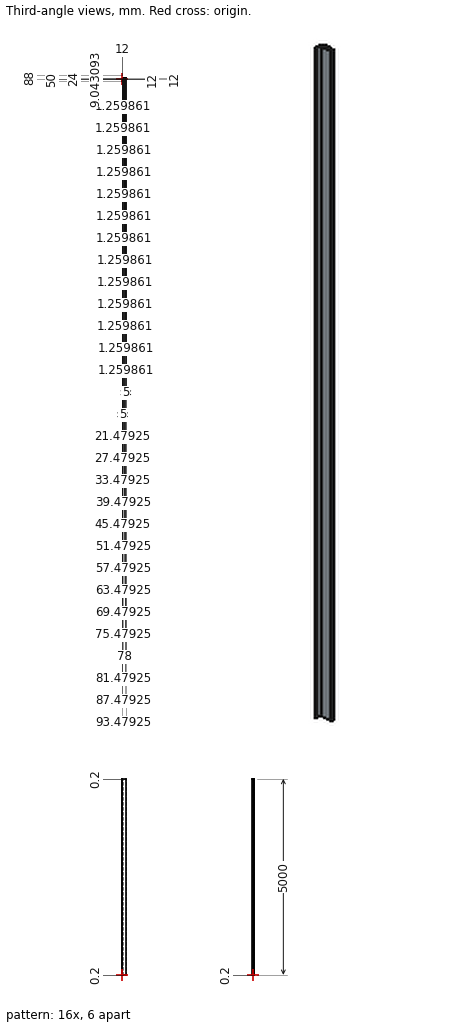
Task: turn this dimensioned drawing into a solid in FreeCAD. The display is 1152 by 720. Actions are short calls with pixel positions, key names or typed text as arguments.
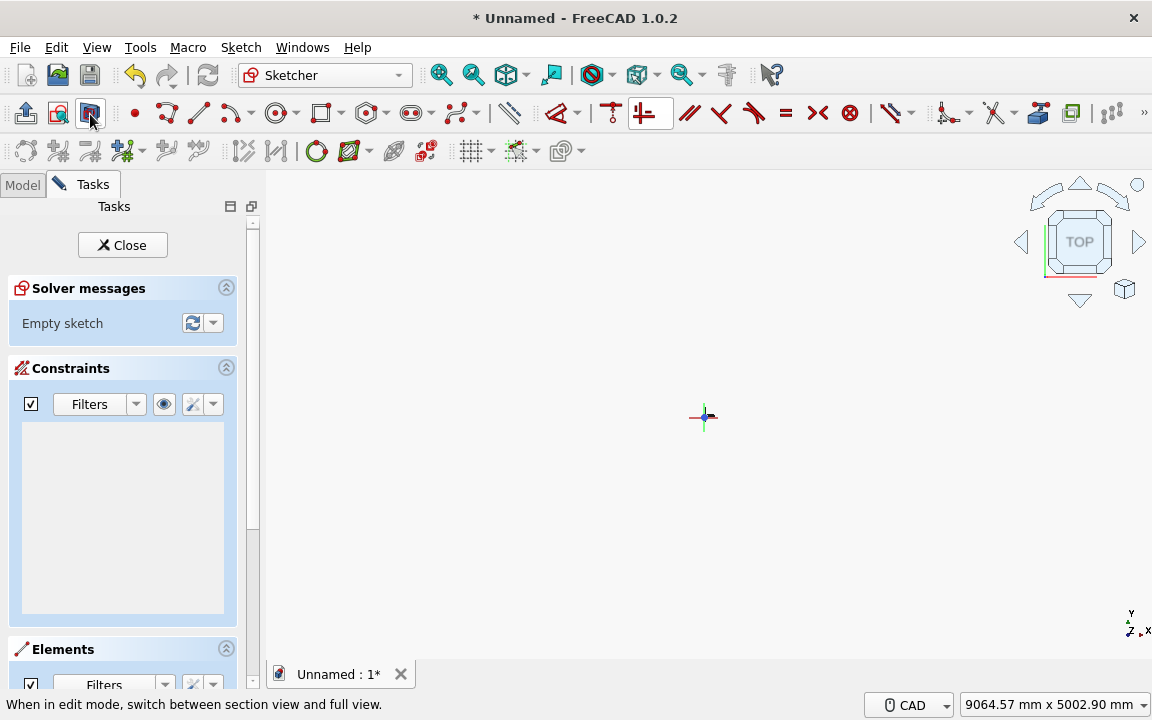
scroll(708, 413, up, 15)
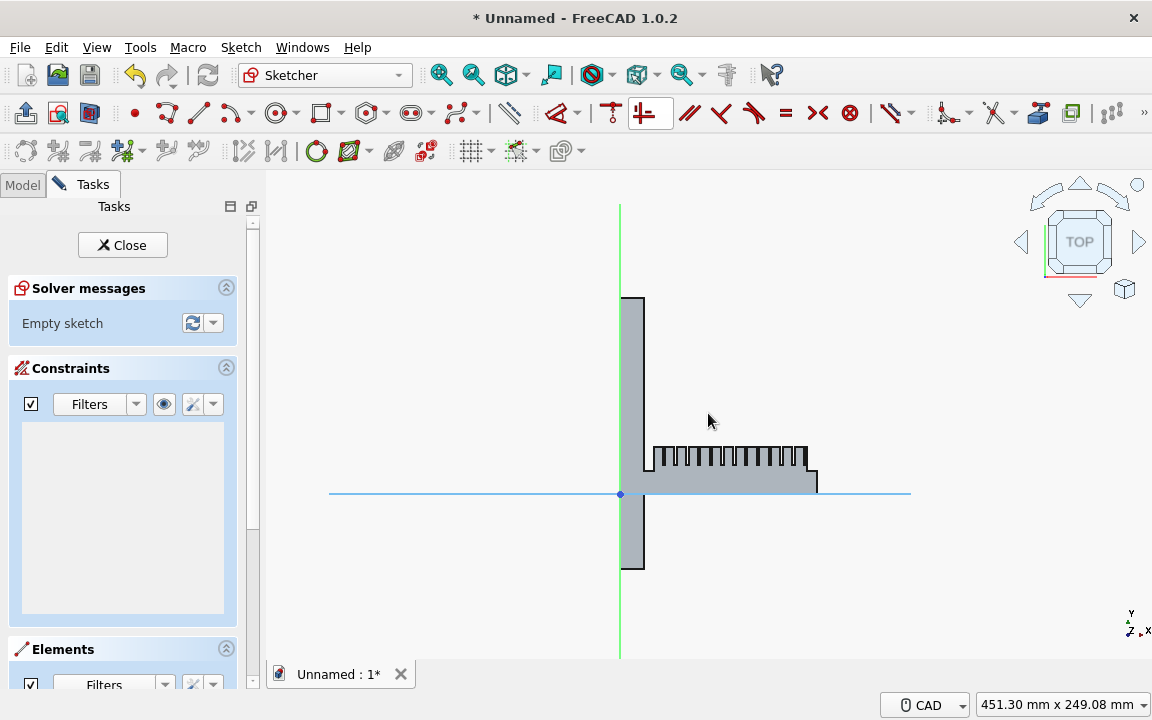
scroll(615, 359, up, 2)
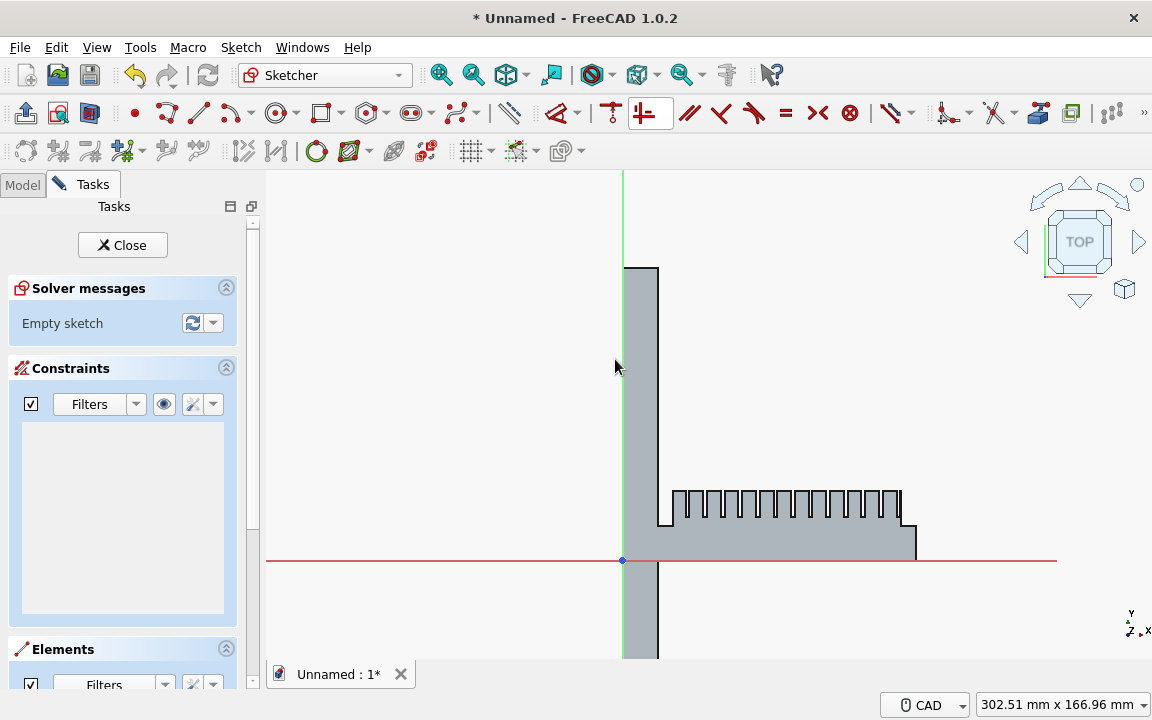
click(322, 114)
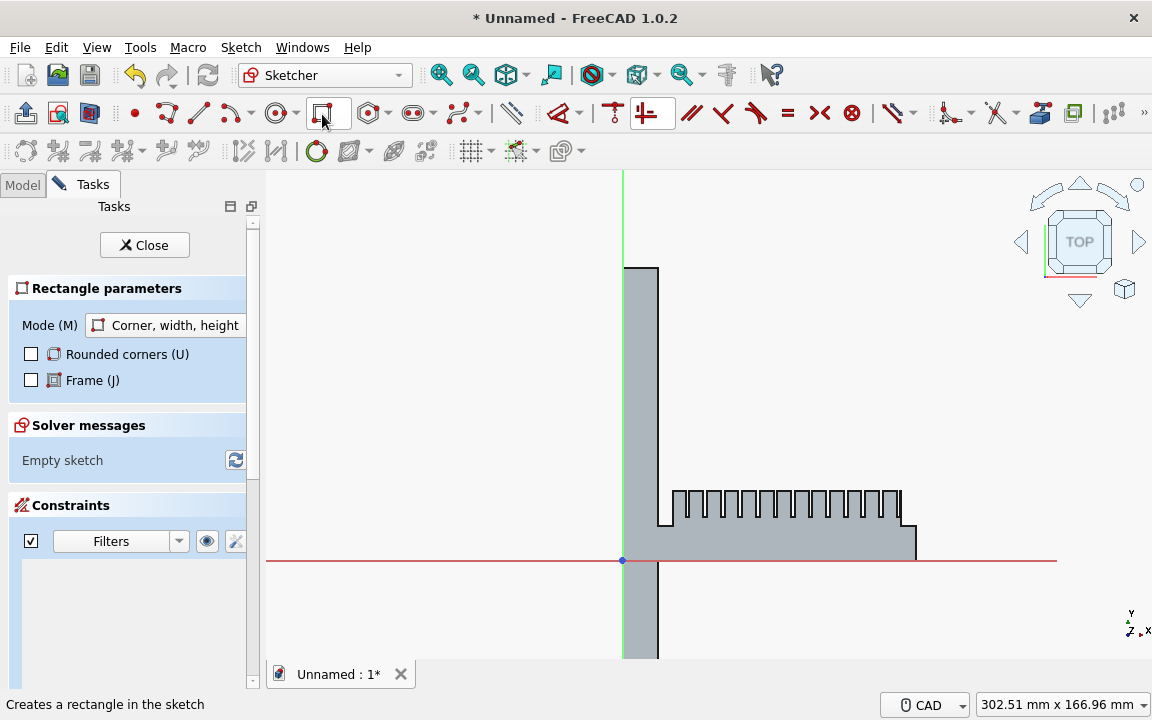
click(623, 268)
click(658, 526)
key(Escape)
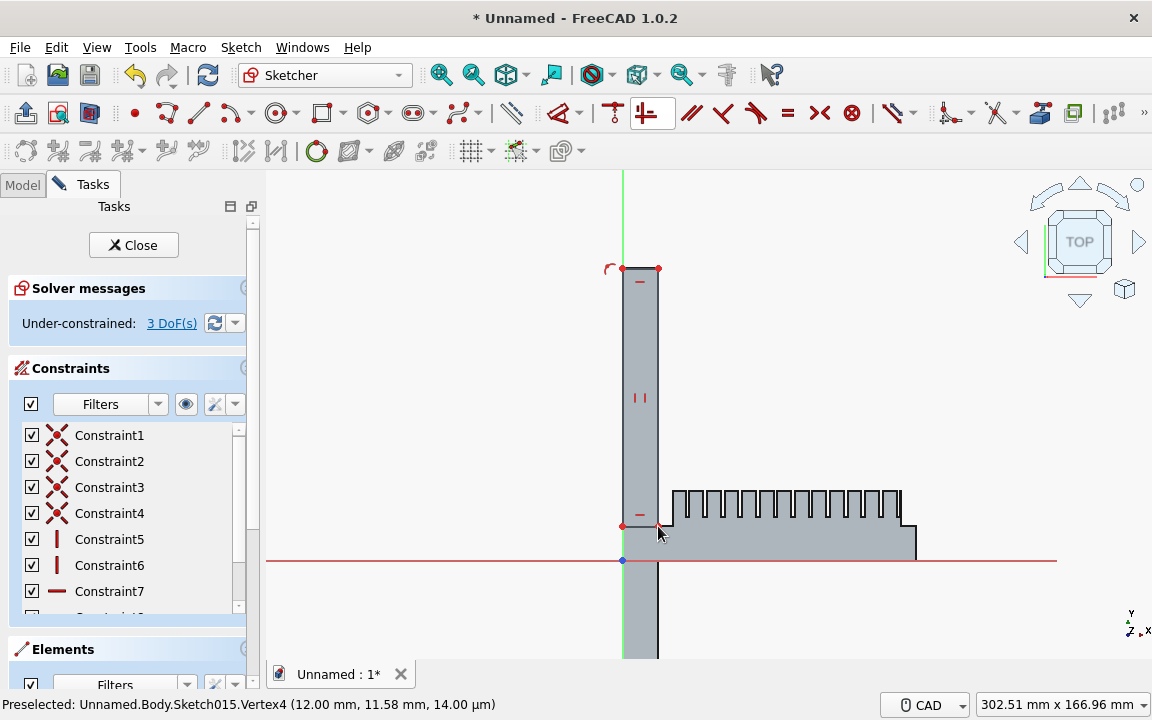
click(558, 114)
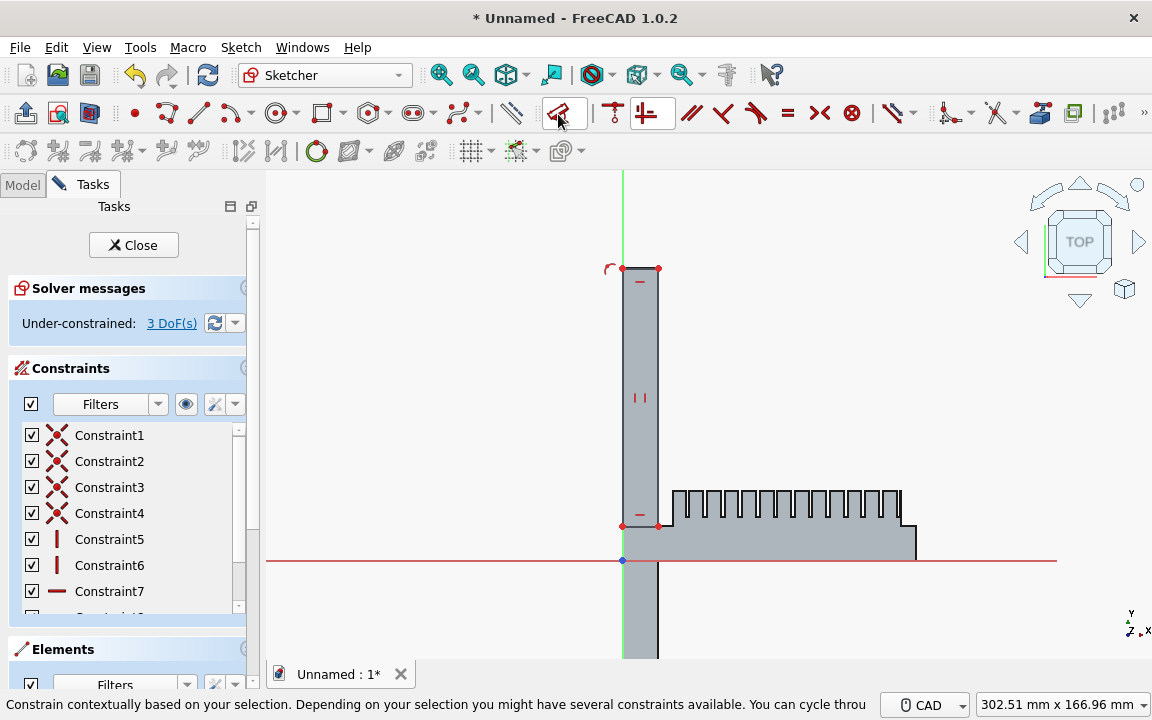
click(623, 346)
click(589, 398)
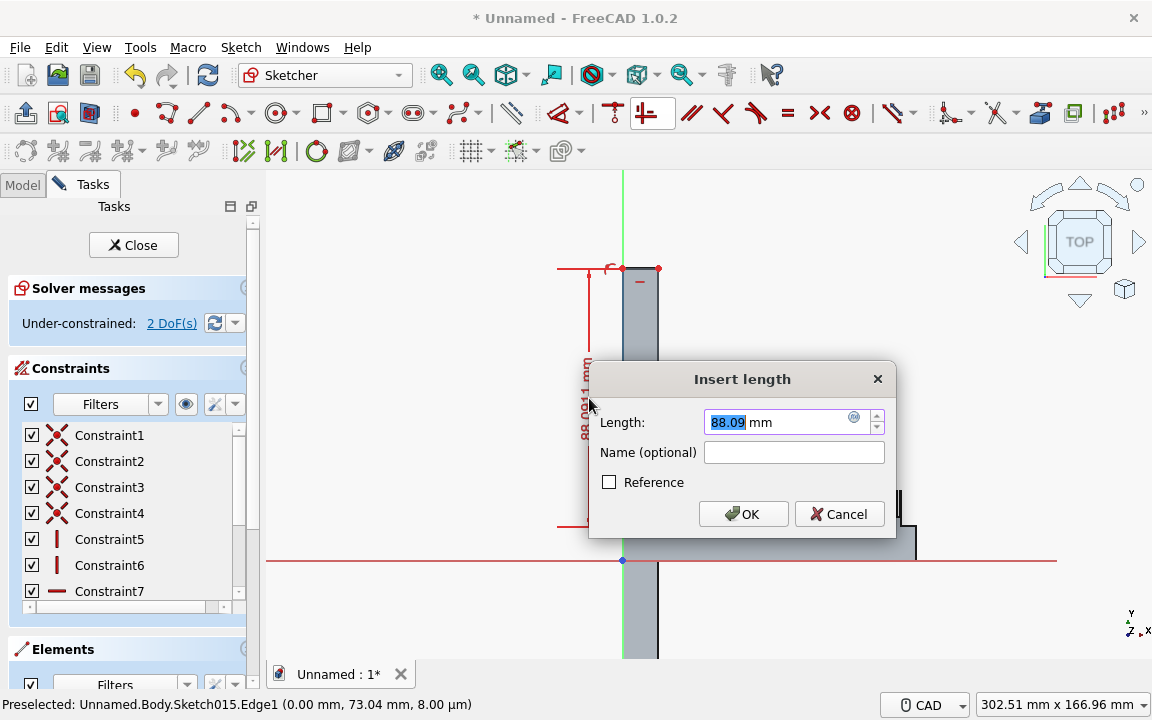
text(88)
key(Return)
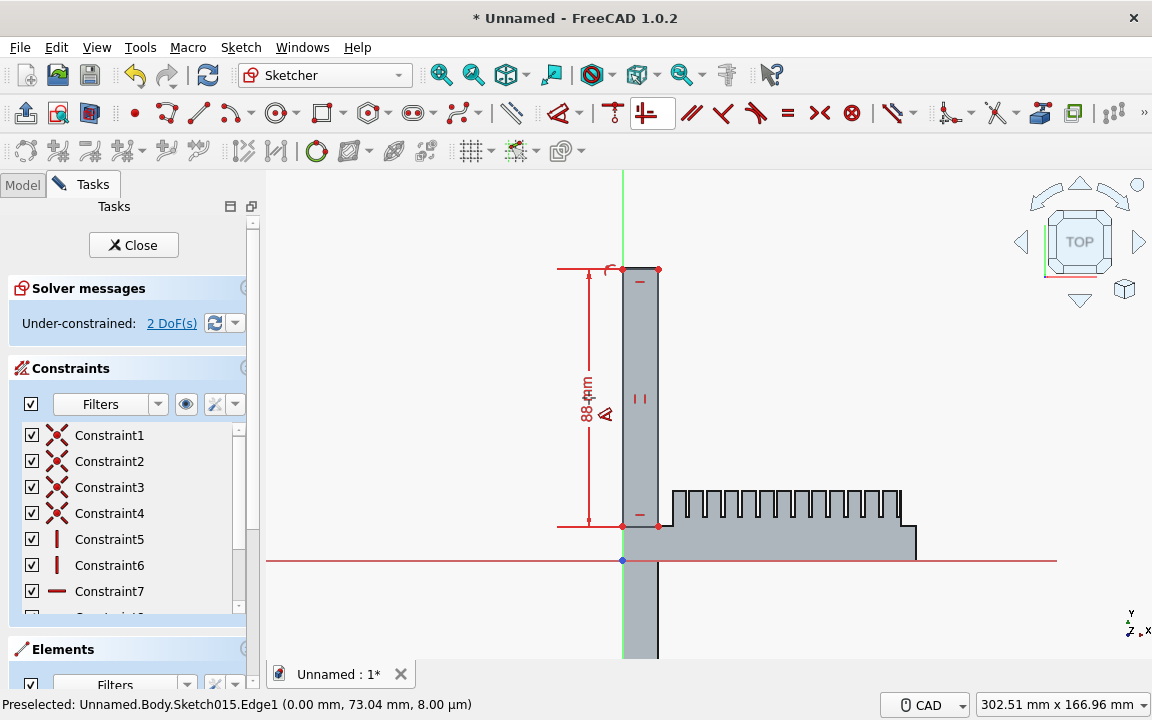
scroll(633, 527, up, 2)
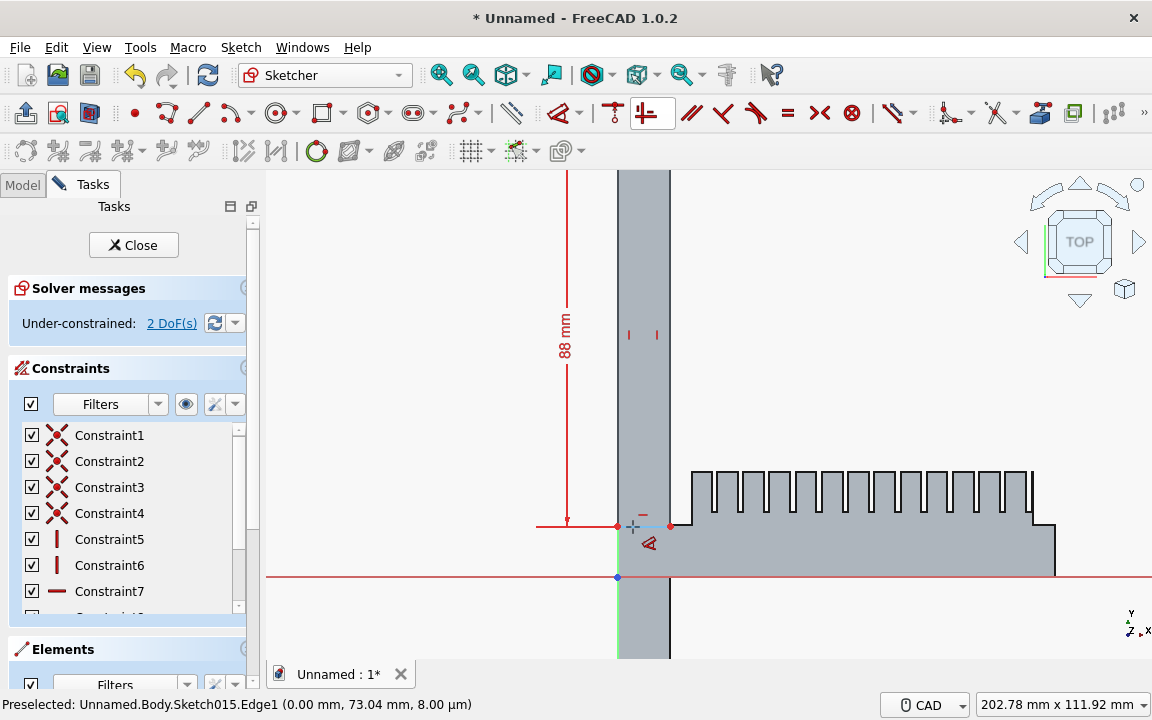
click(633, 527)
click(644, 561)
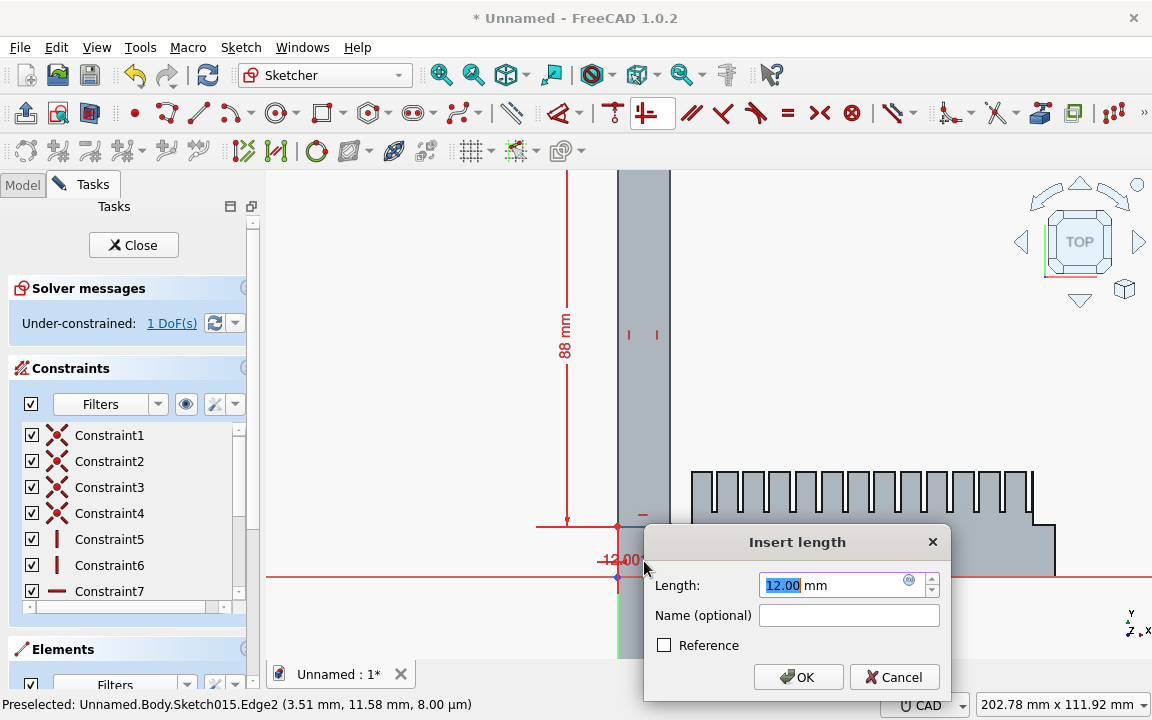
text(12)
key(Return)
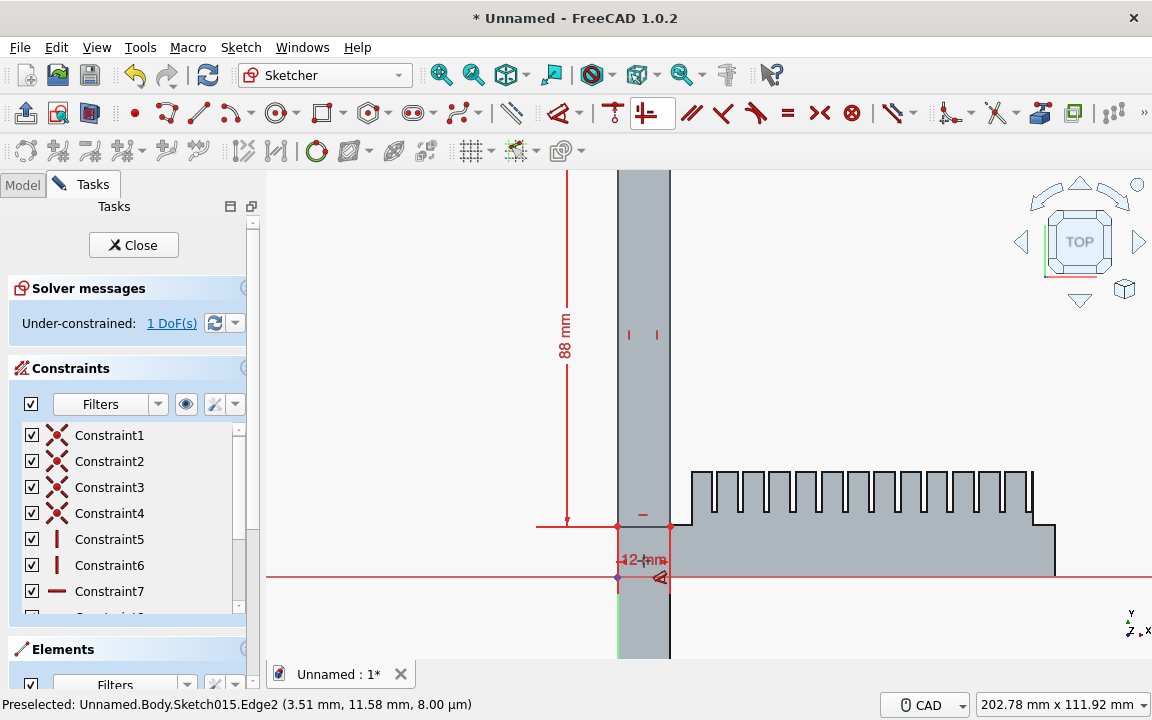
click(618, 527)
click(584, 540)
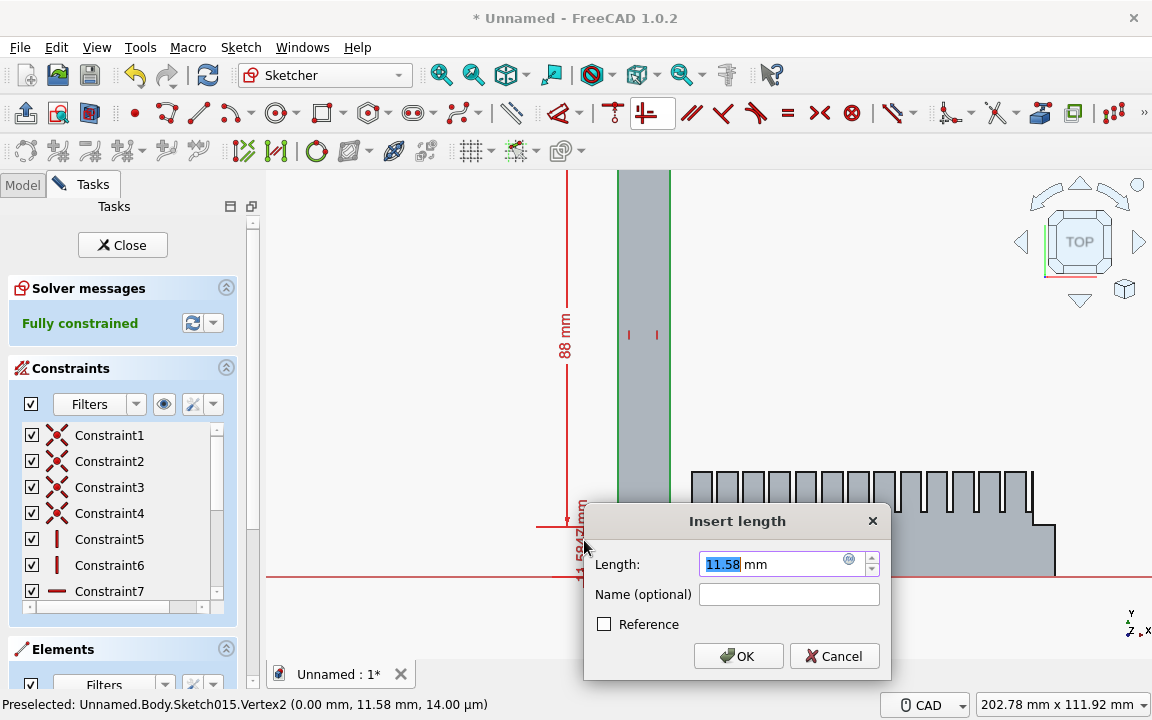
text(12)
key(Return)
key(Escape)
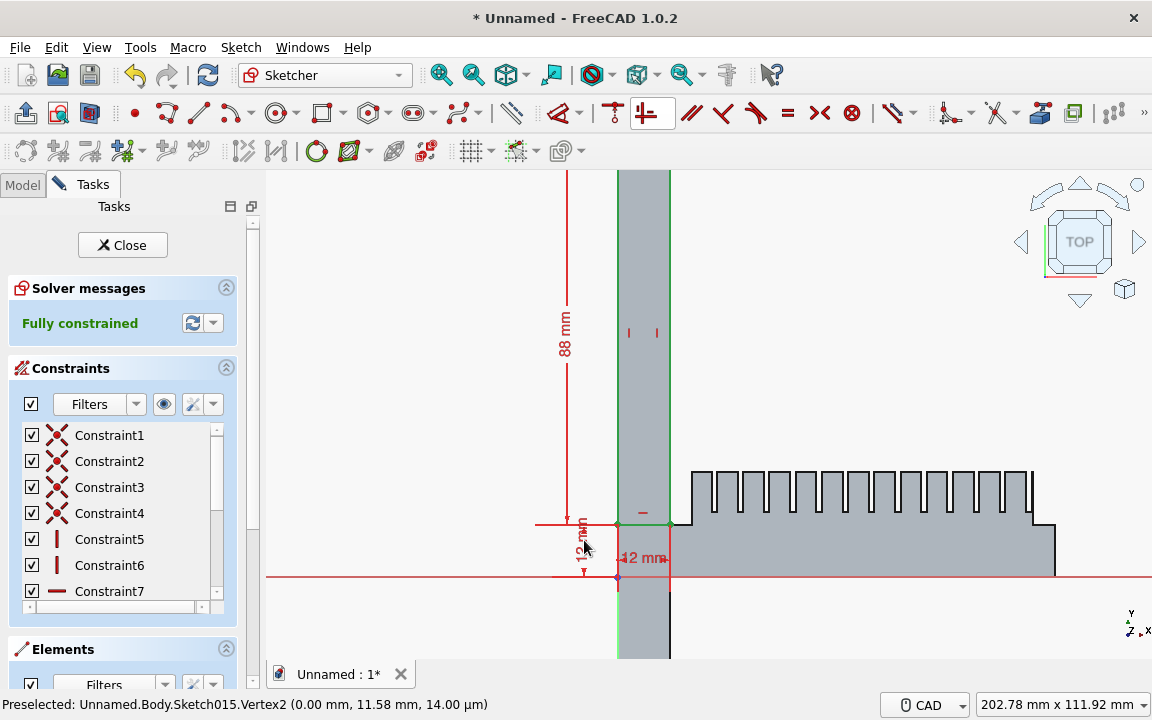
click(123, 245)